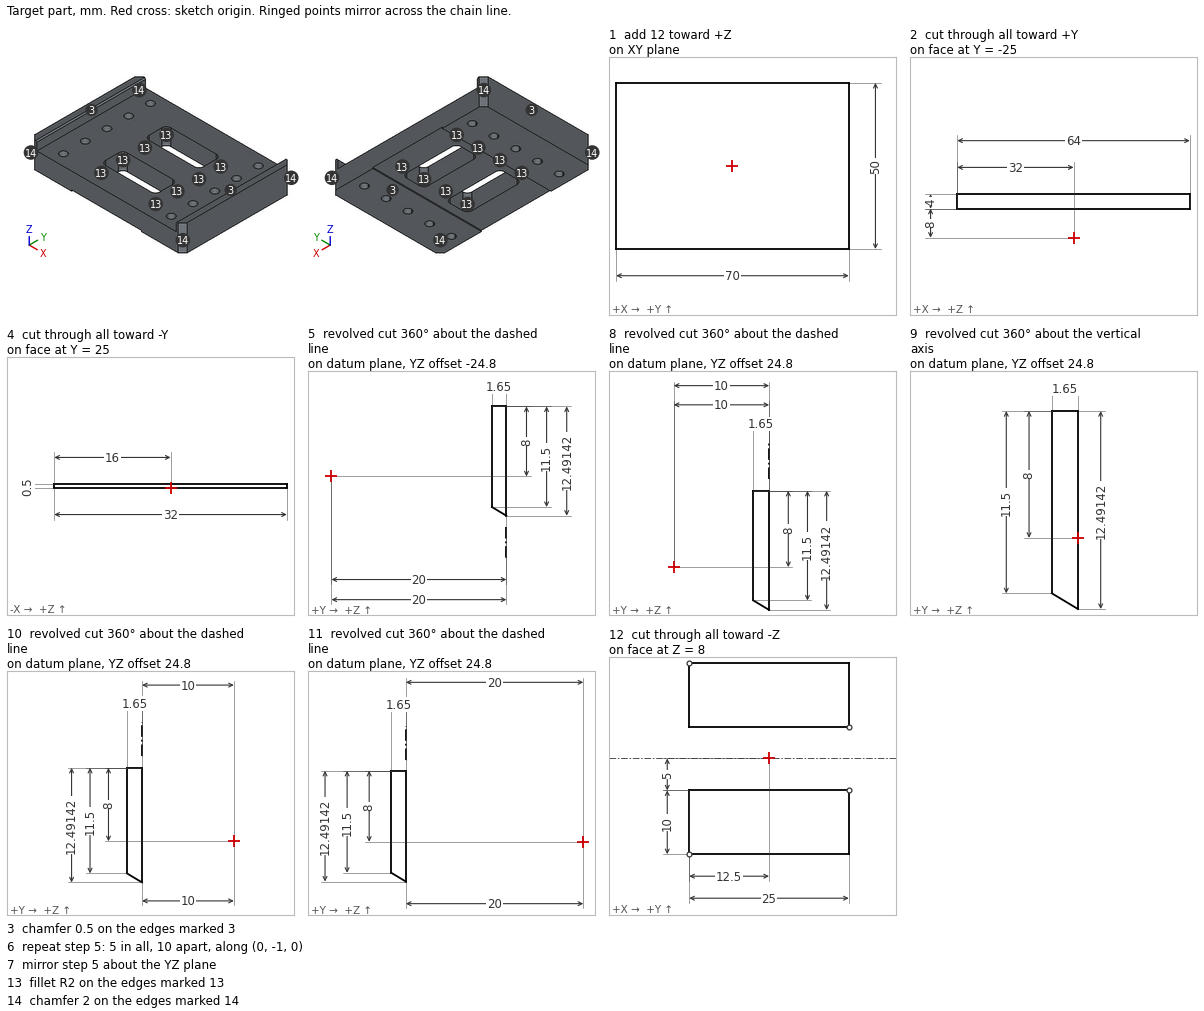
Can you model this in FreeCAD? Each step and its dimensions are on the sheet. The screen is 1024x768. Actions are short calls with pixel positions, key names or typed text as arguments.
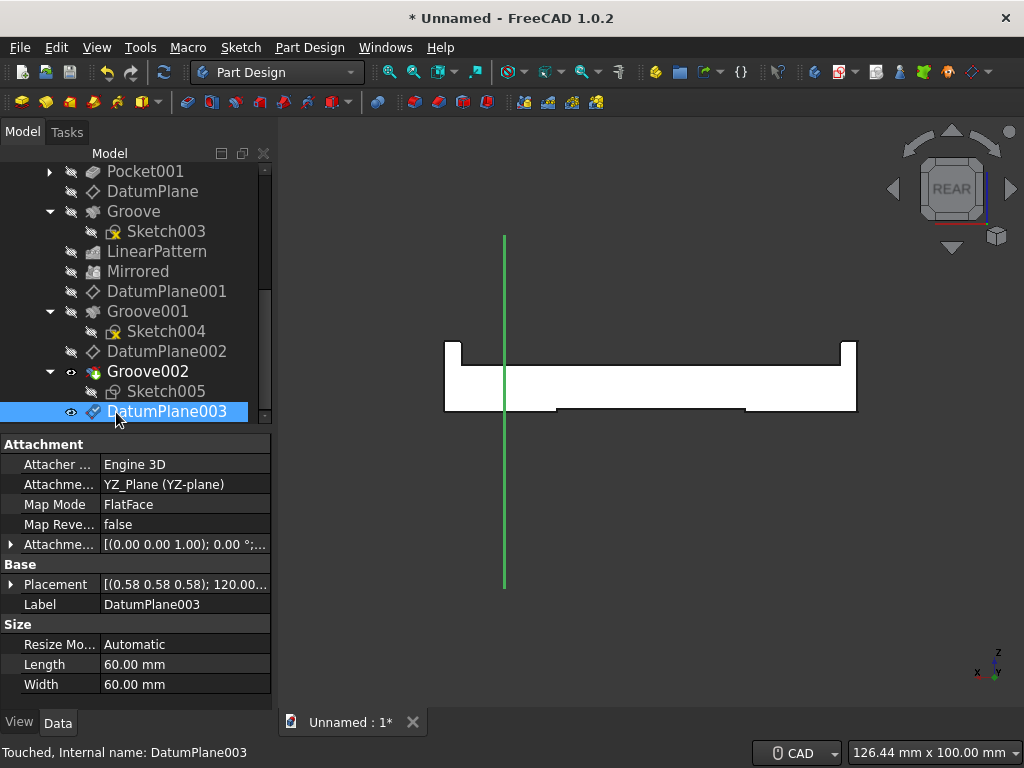
click(840, 72)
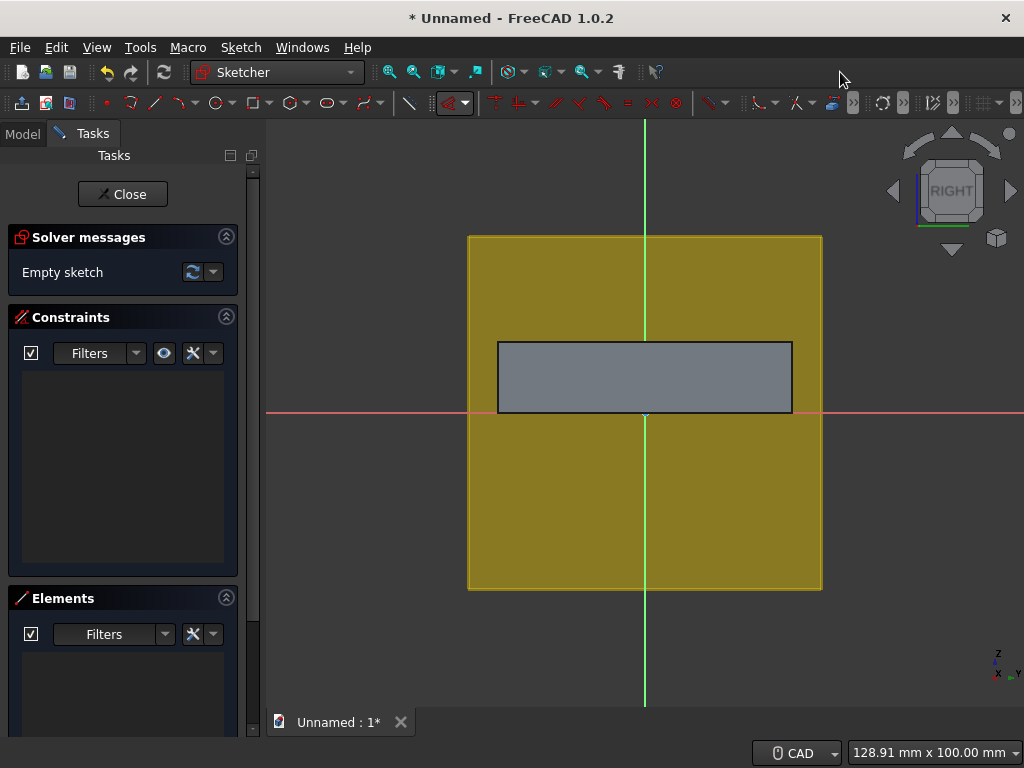
key(q)
key(s)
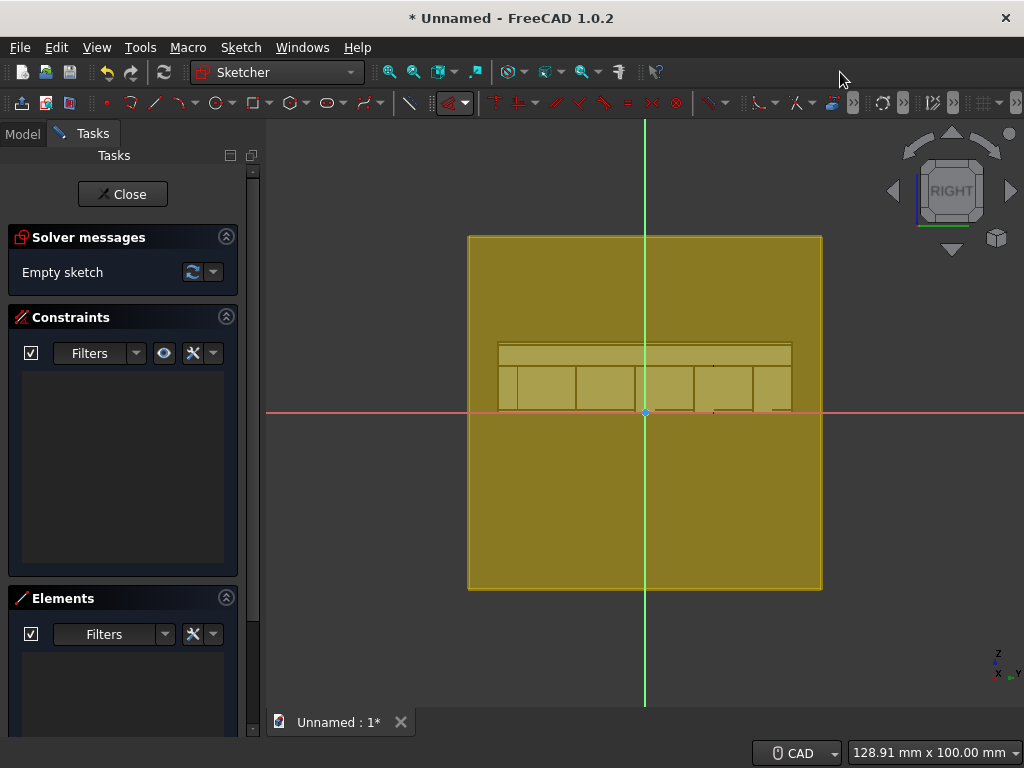
scroll(626, 377, up, 6)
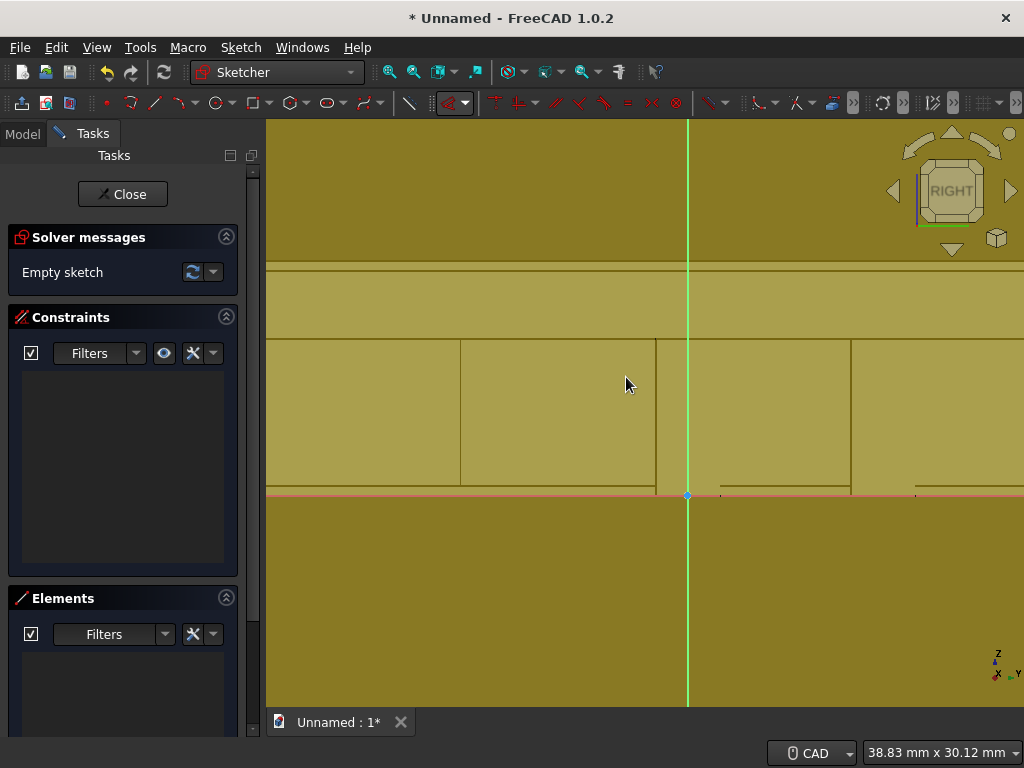
click(132, 104)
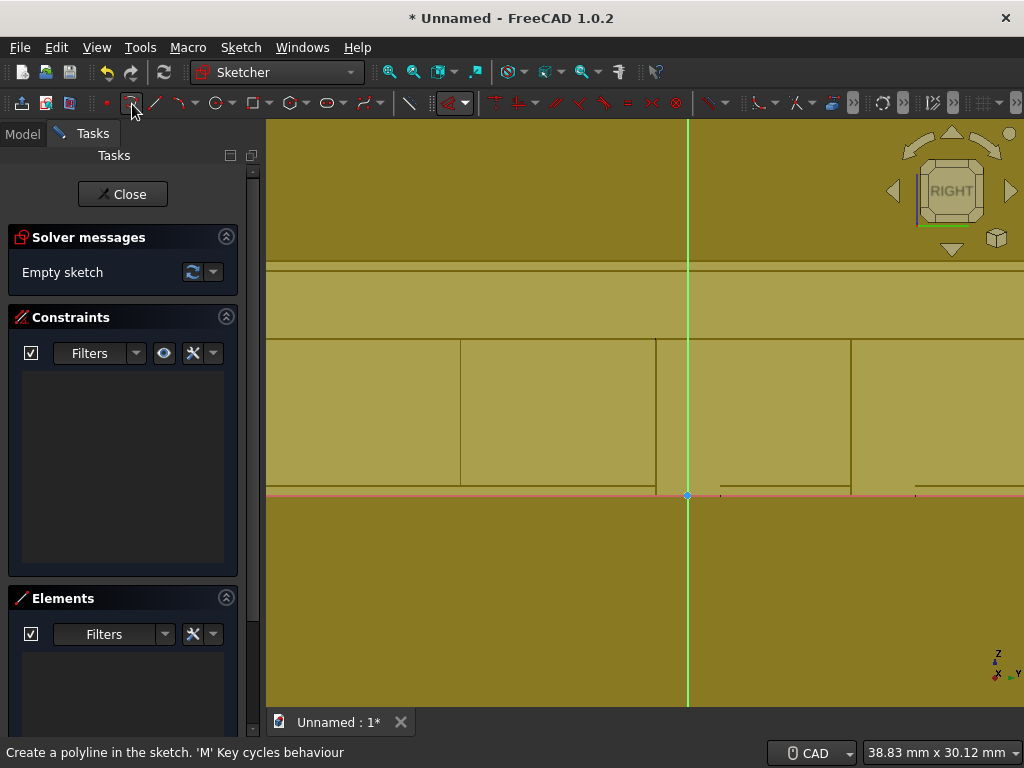
click(493, 583)
click(461, 564)
click(461, 339)
click(493, 339)
click(493, 584)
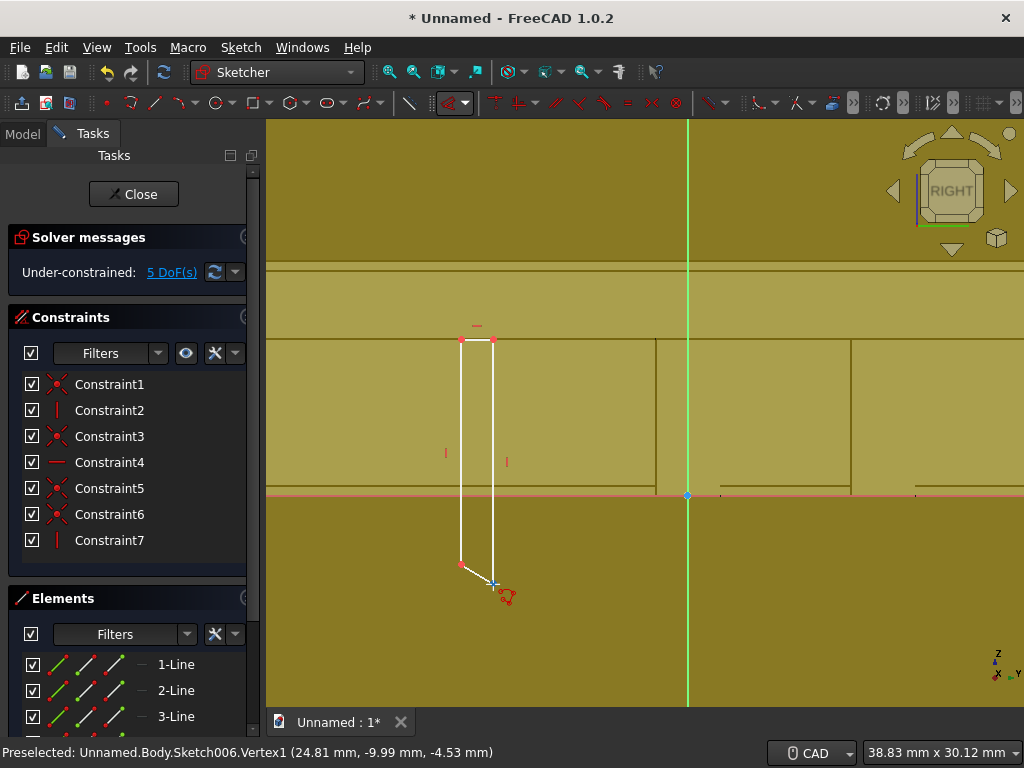
key(g)
key(l)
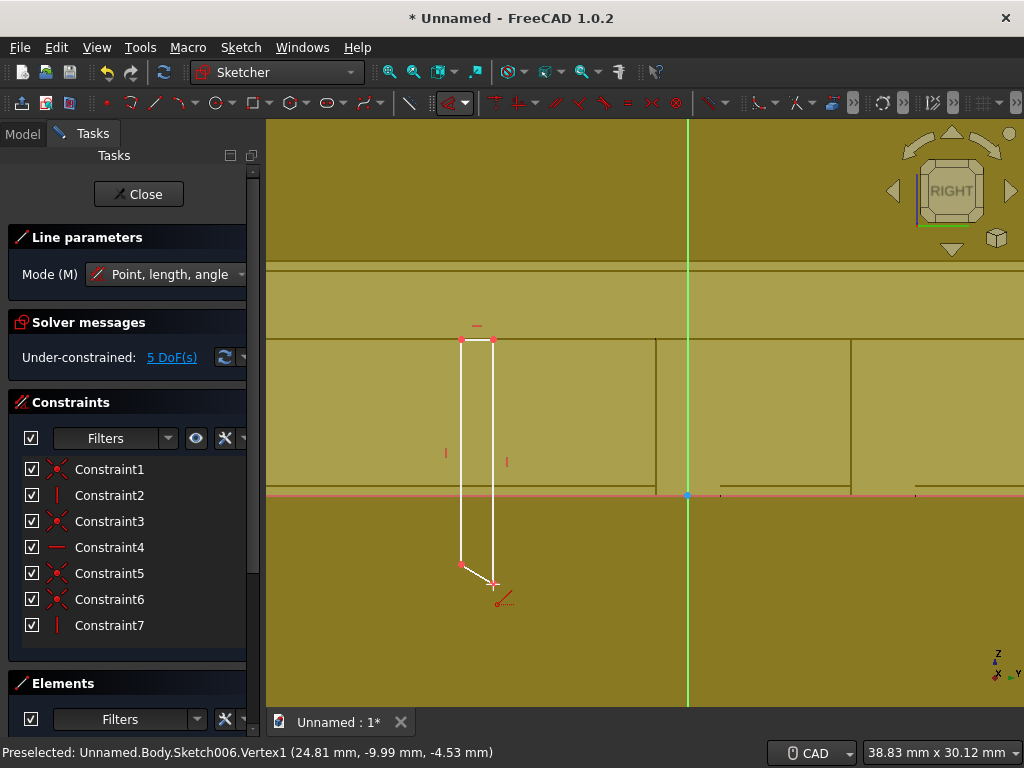
click(493, 315)
click(493, 242)
key(Escape)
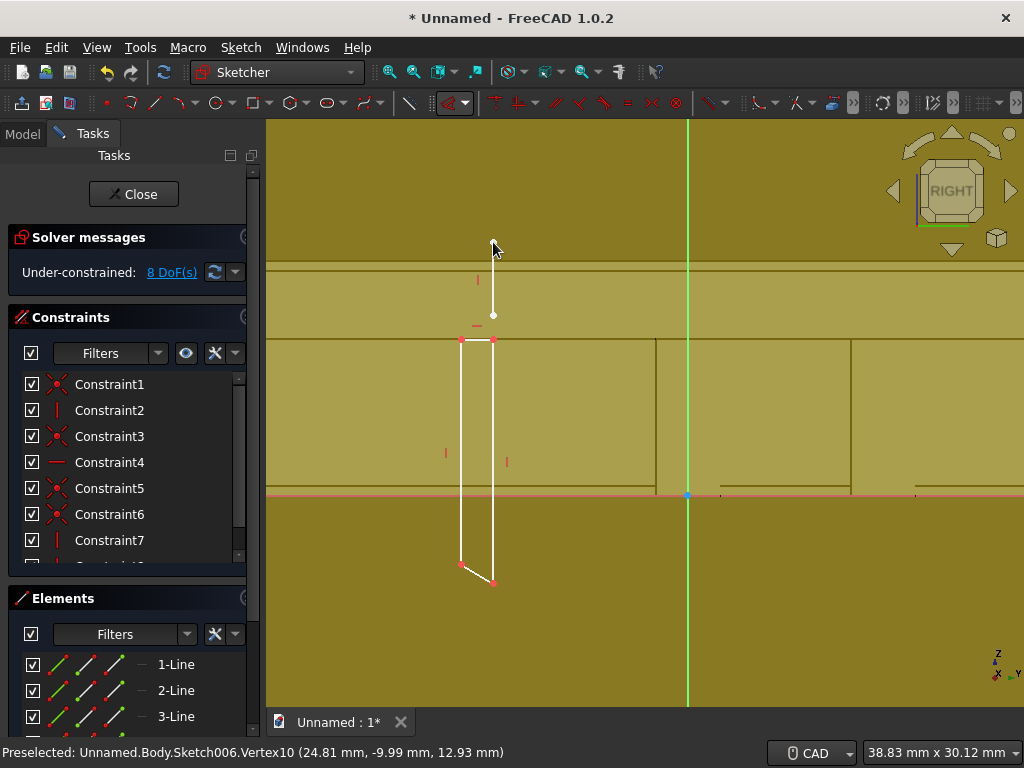
click(493, 294)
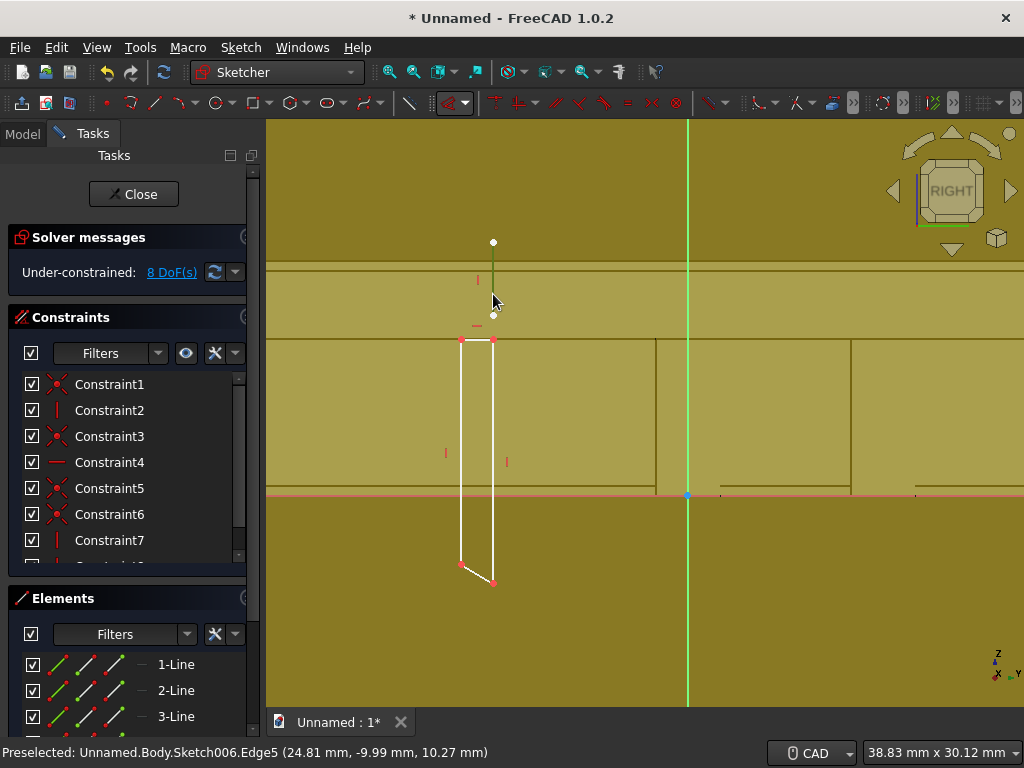
key(g)
key(n)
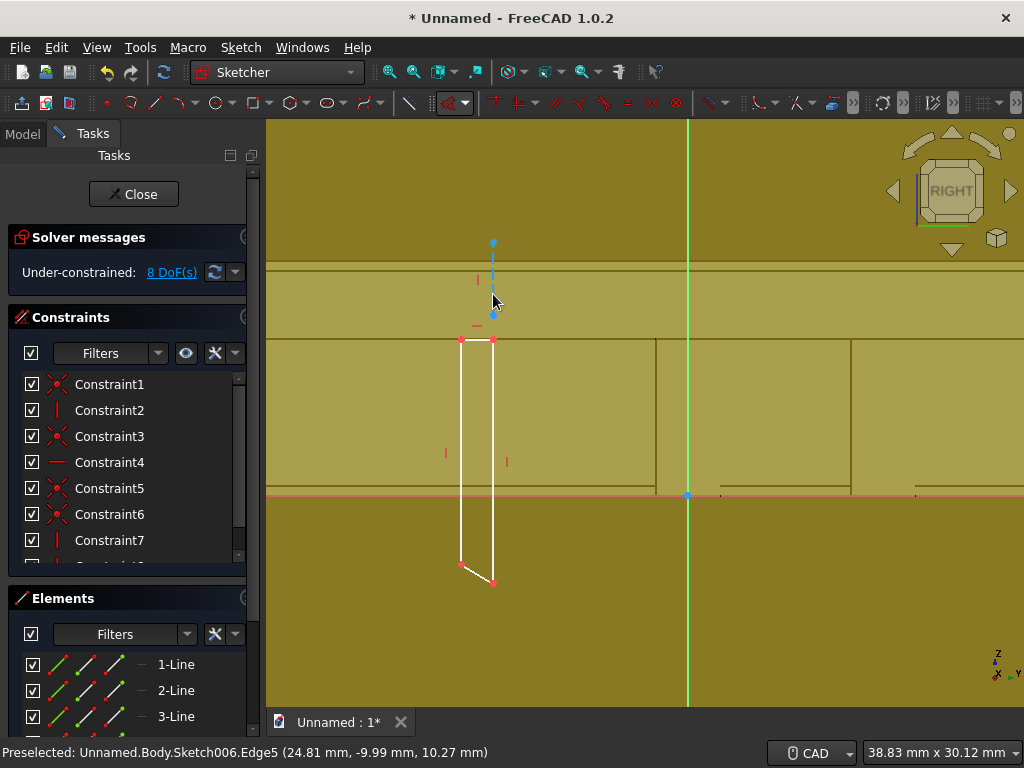
click(461, 340)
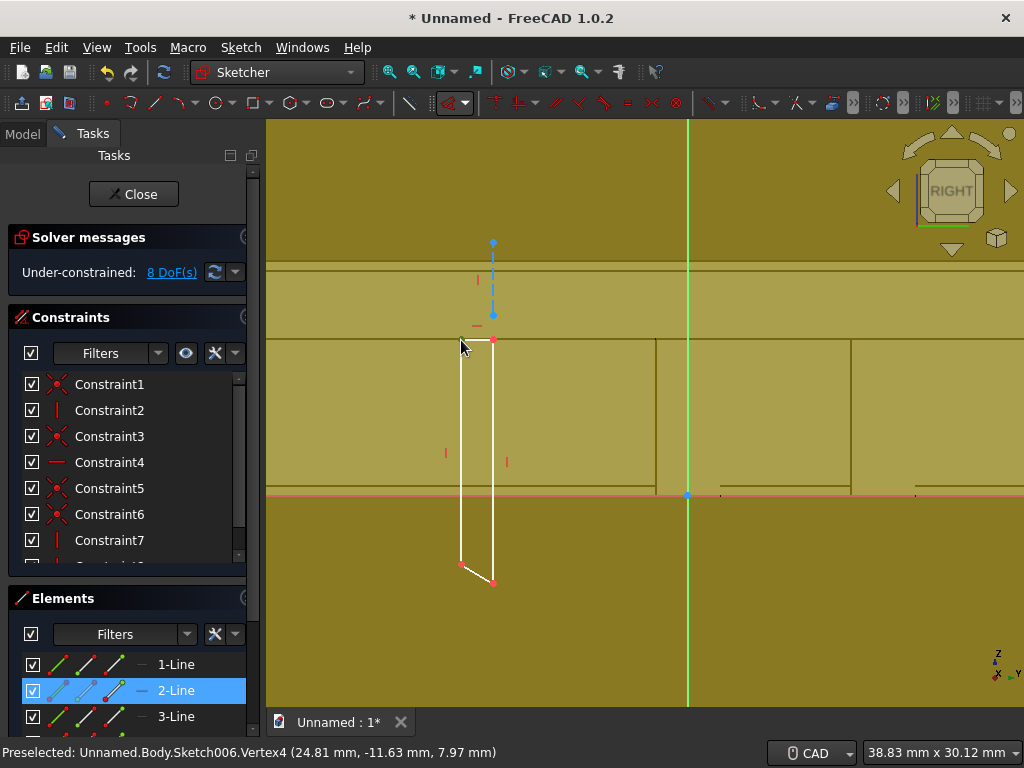
key(i)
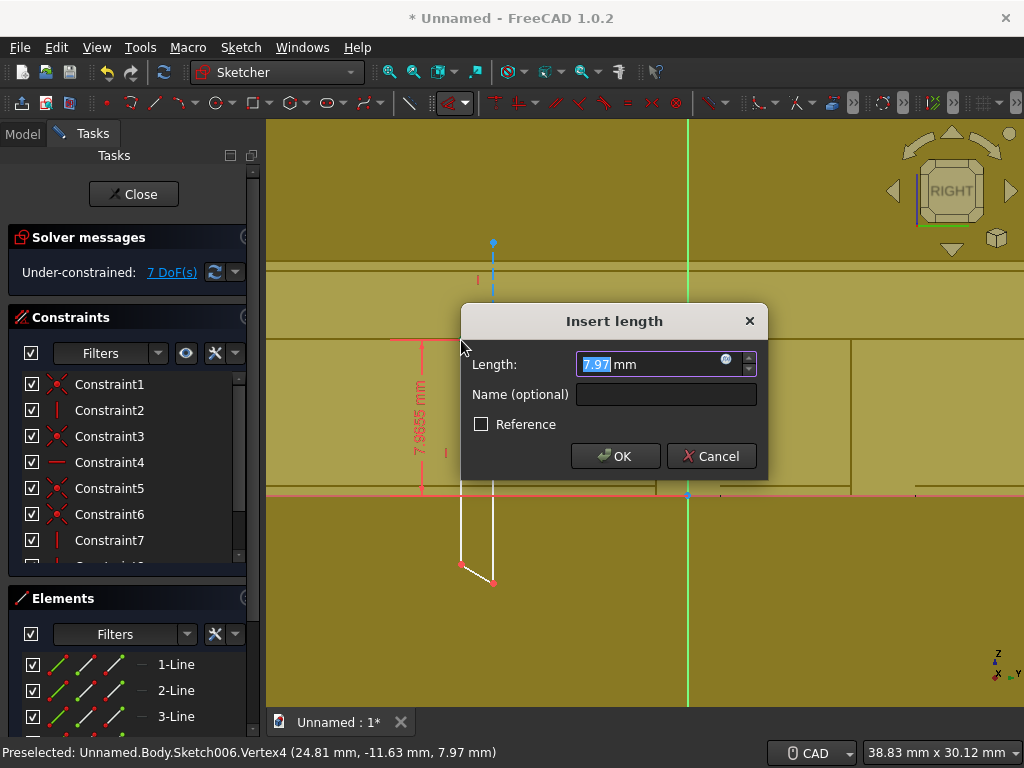
text(8)
key(Return)